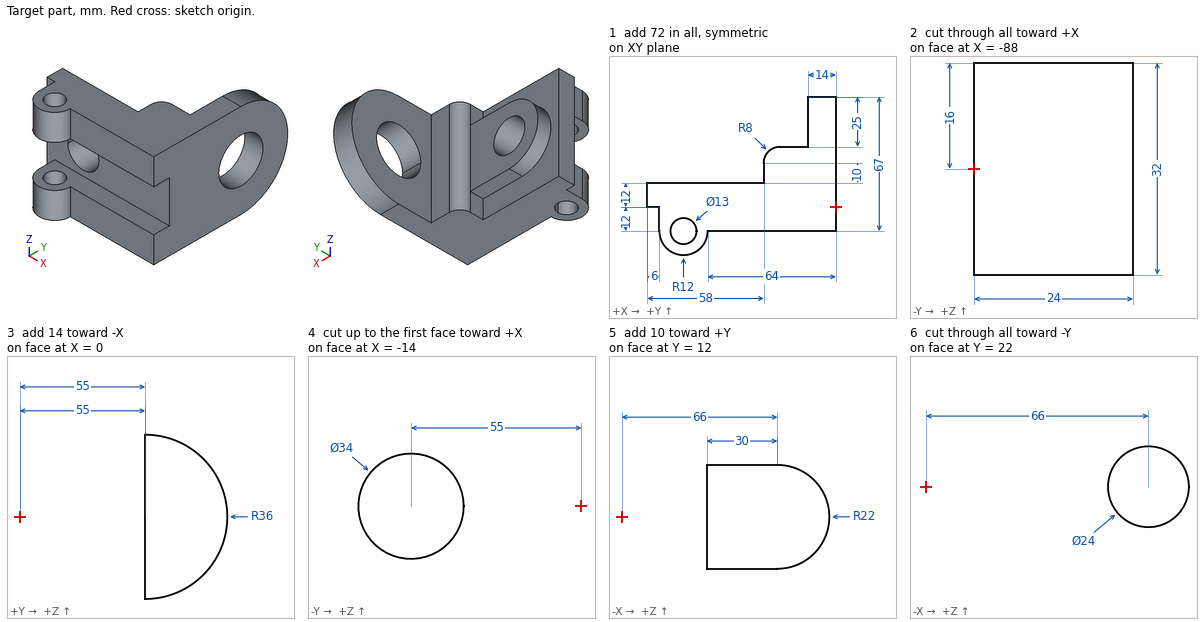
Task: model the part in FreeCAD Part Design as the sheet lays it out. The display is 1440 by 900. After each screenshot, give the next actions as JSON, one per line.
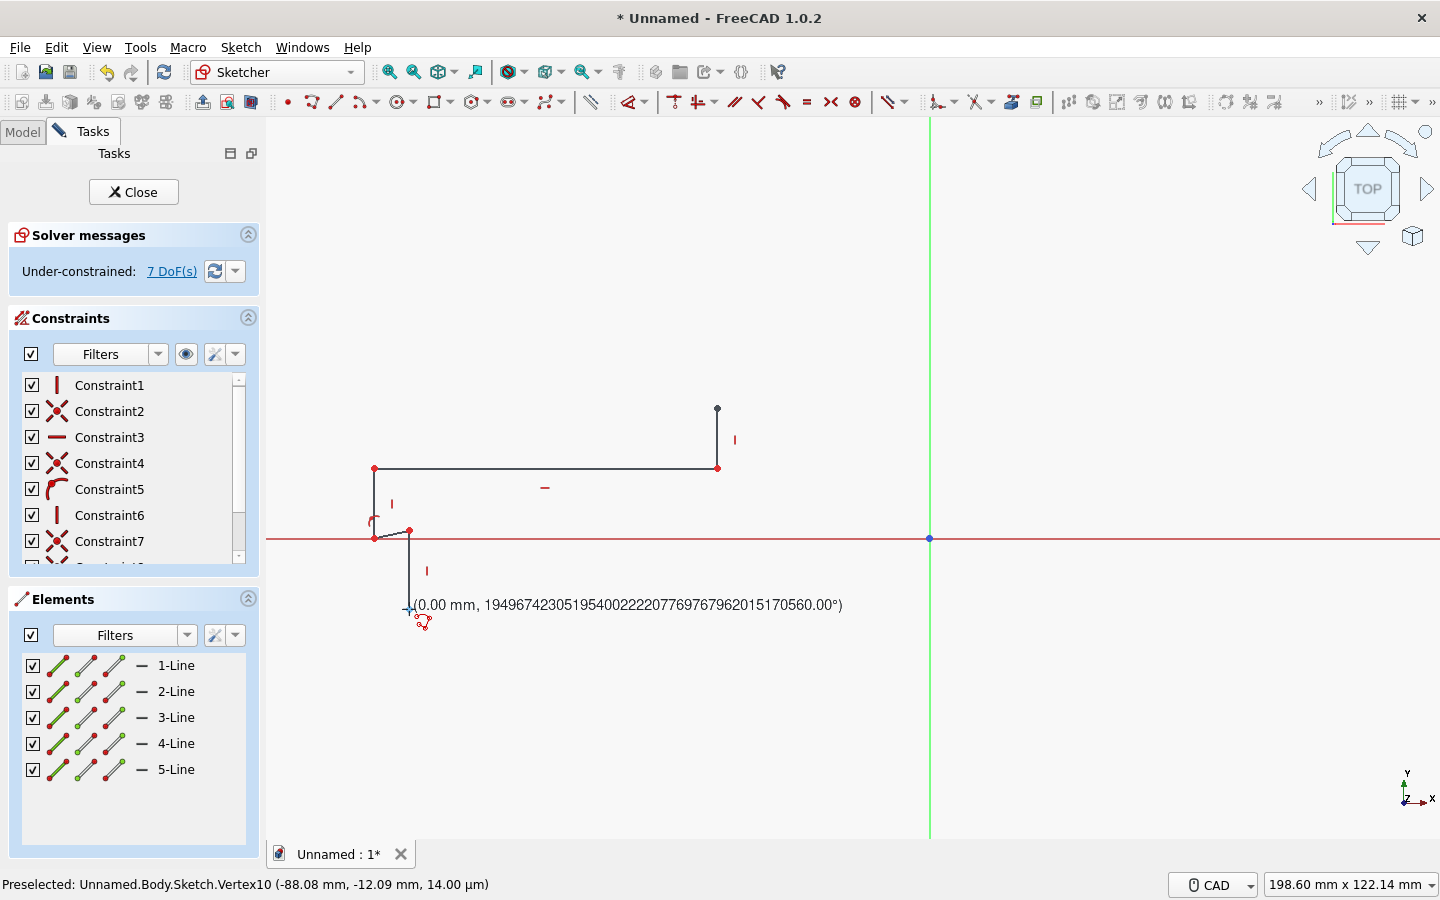
{"action": "left_click", "coordinate": [551, 609]}
{"action": "left_click", "coordinate": [930, 609]}
{"action": "left_click", "coordinate": [921, 213]}
{"action": "left_click", "coordinate": [847, 213]}
{"action": "left_click", "coordinate": [847, 361]}
{"action": "left_click", "coordinate": [764, 361]}
{"action": "right_click", "coordinate": [764, 361]}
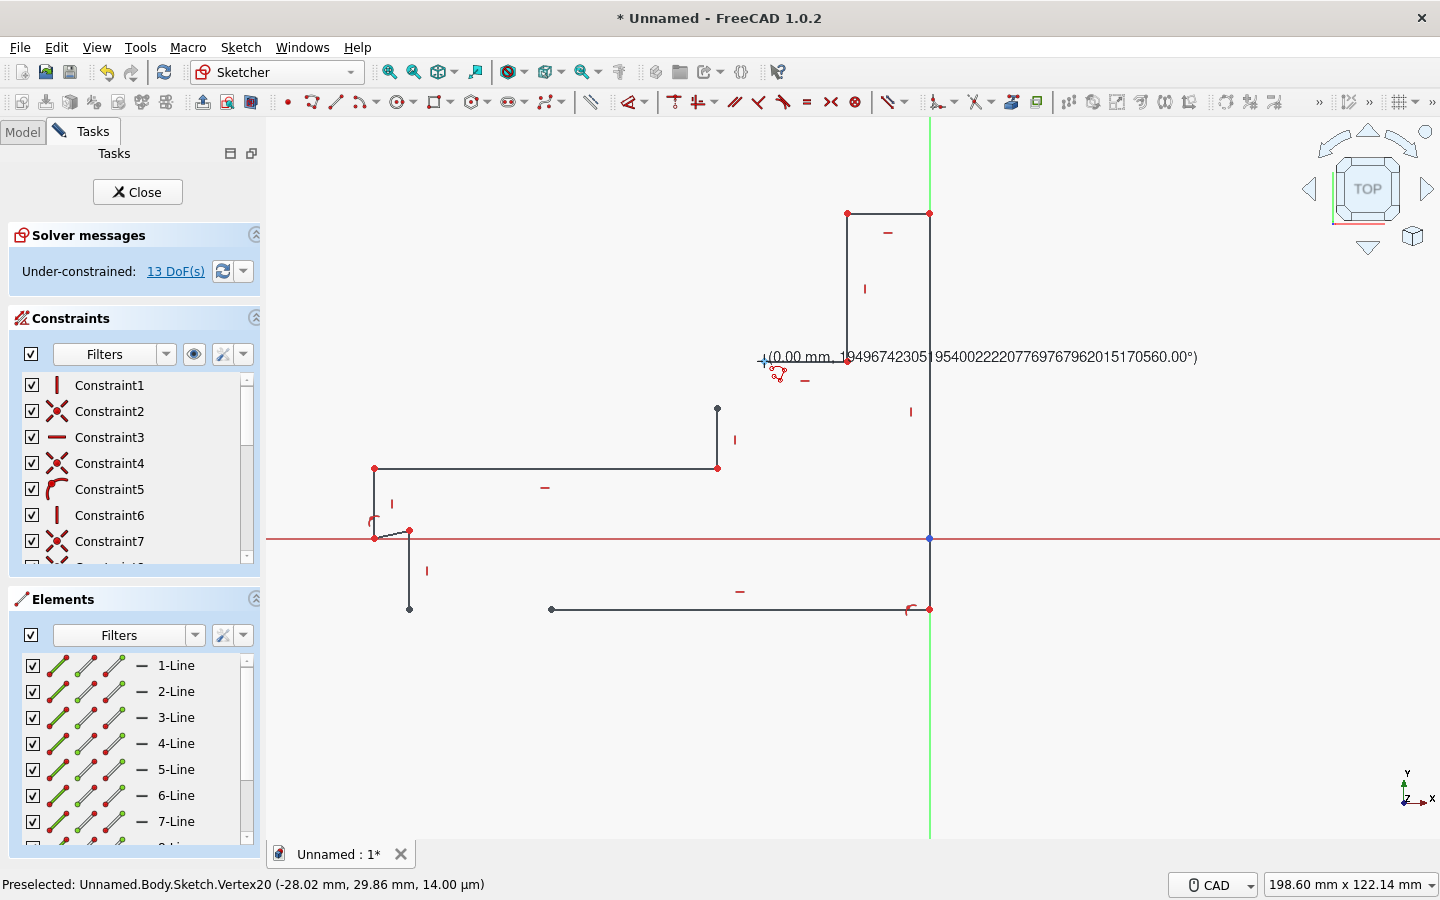
{"action": "left_click", "coordinate": [378, 102]}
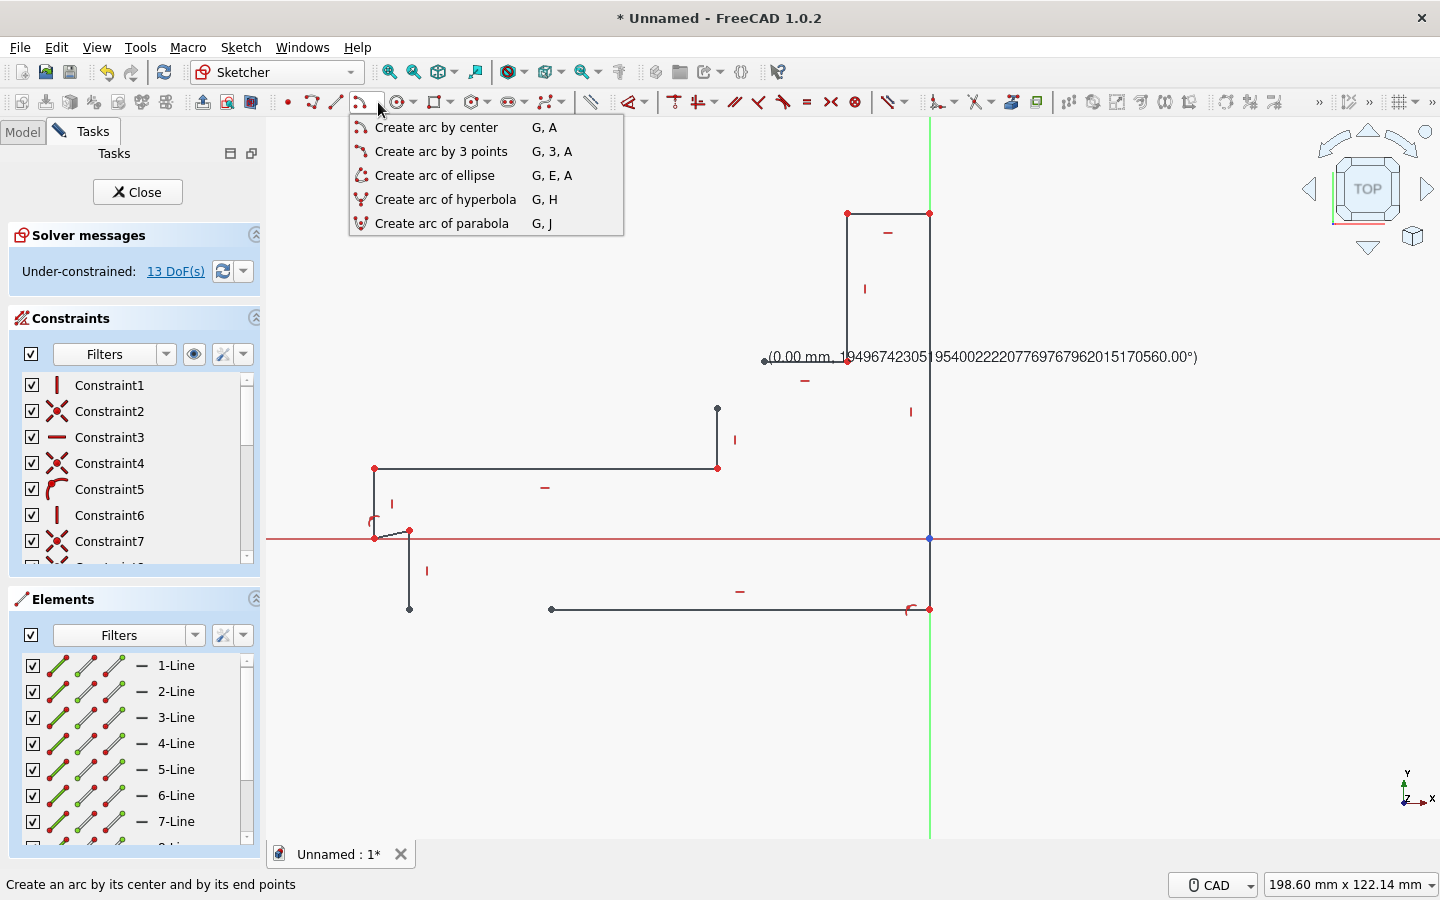
{"action": "left_click", "coordinate": [486, 151]}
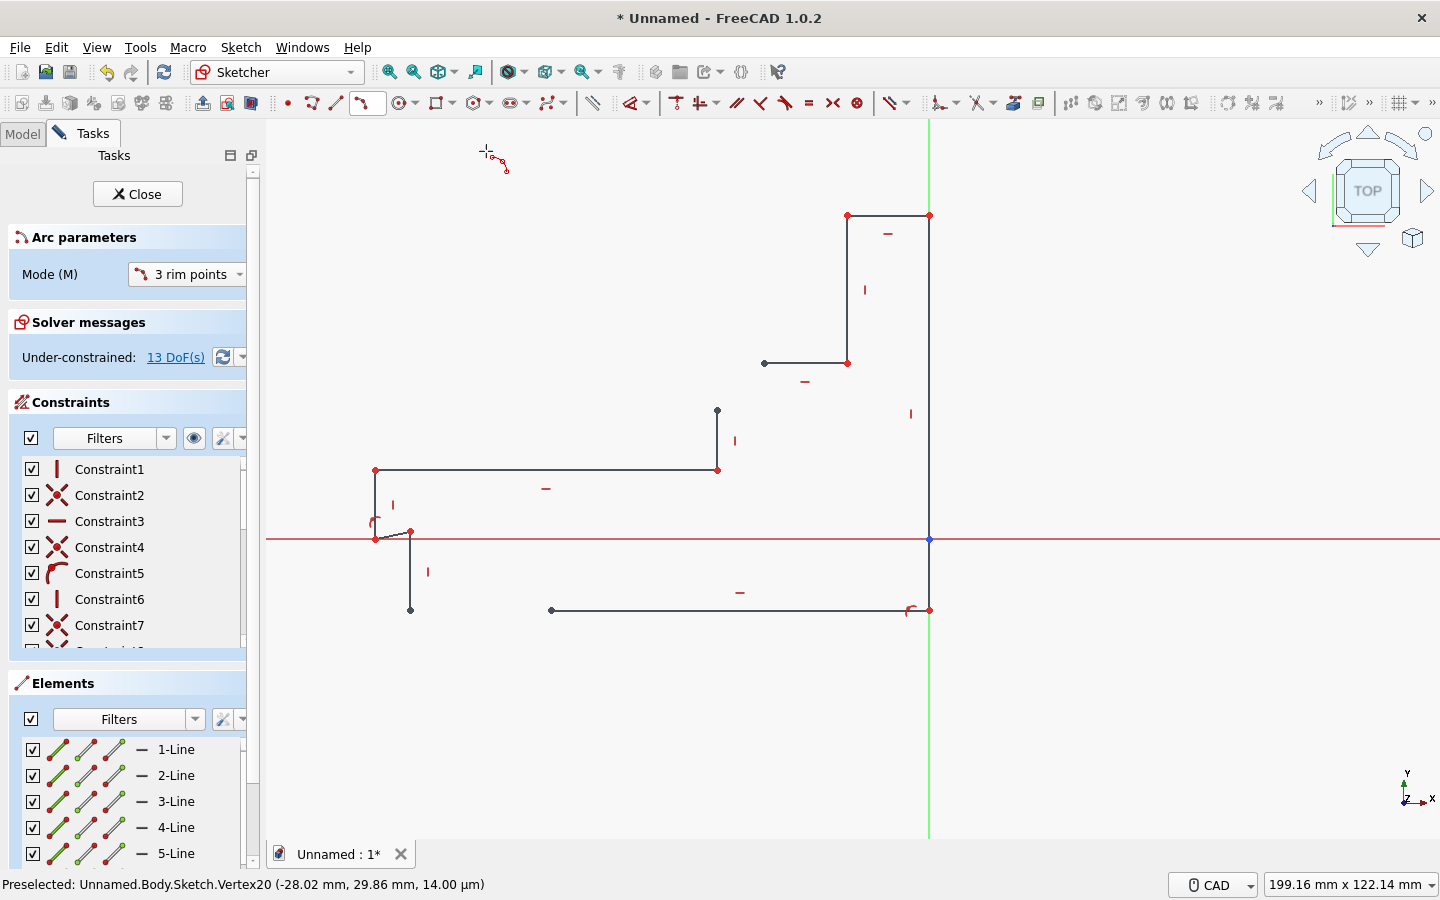
{"action": "left_click", "coordinate": [410, 611]}
{"action": "left_click", "coordinate": [552, 611]}
{"action": "left_click", "coordinate": [481, 681]}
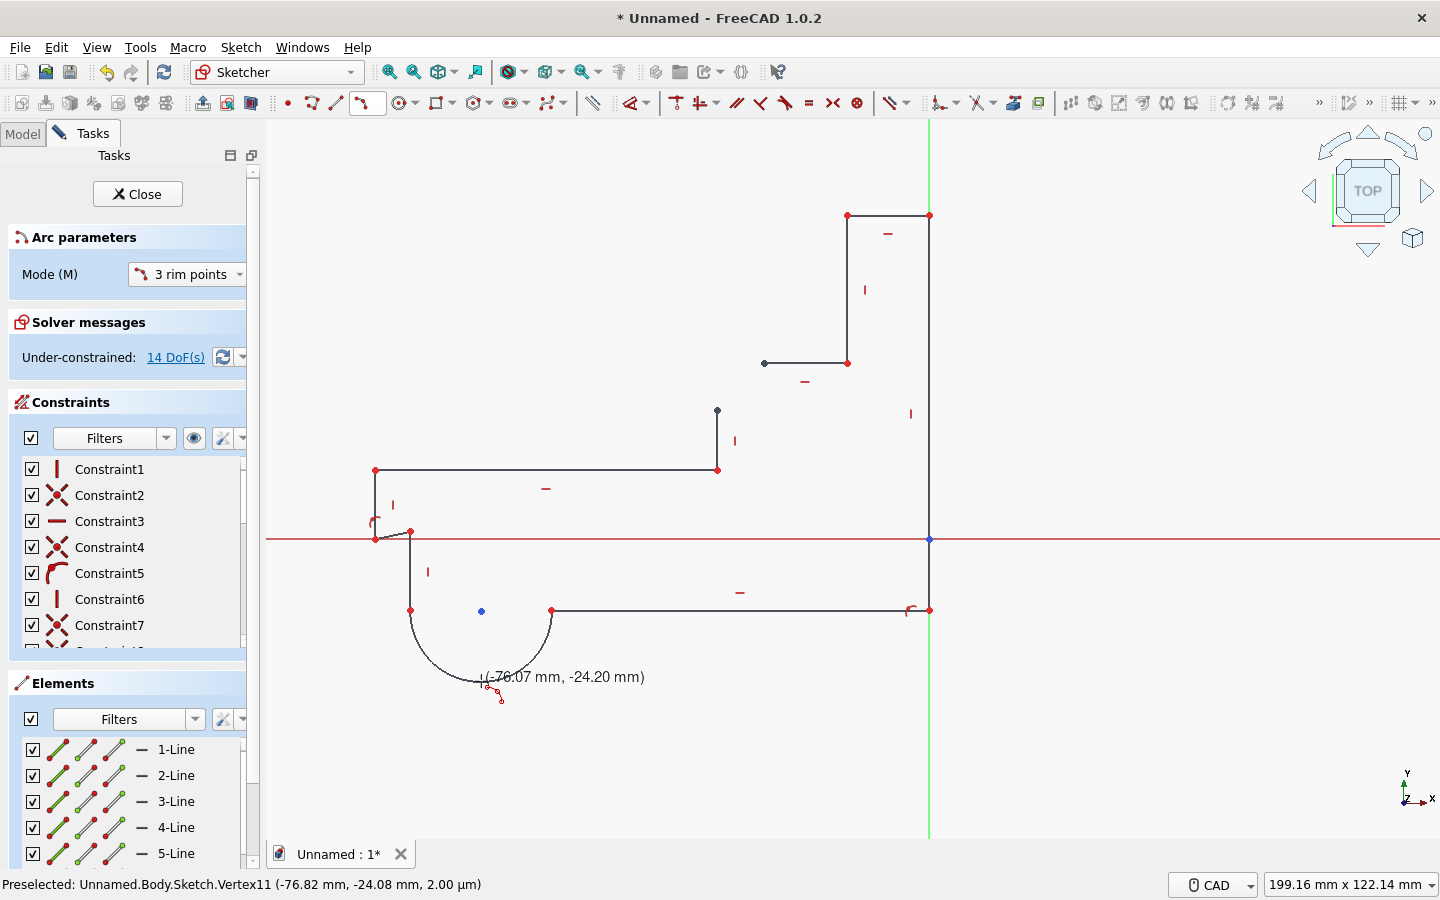
{"action": "left_click", "coordinate": [764, 363]}
{"action": "left_click", "coordinate": [717, 410]}
{"action": "left_click", "coordinate": [731, 376]}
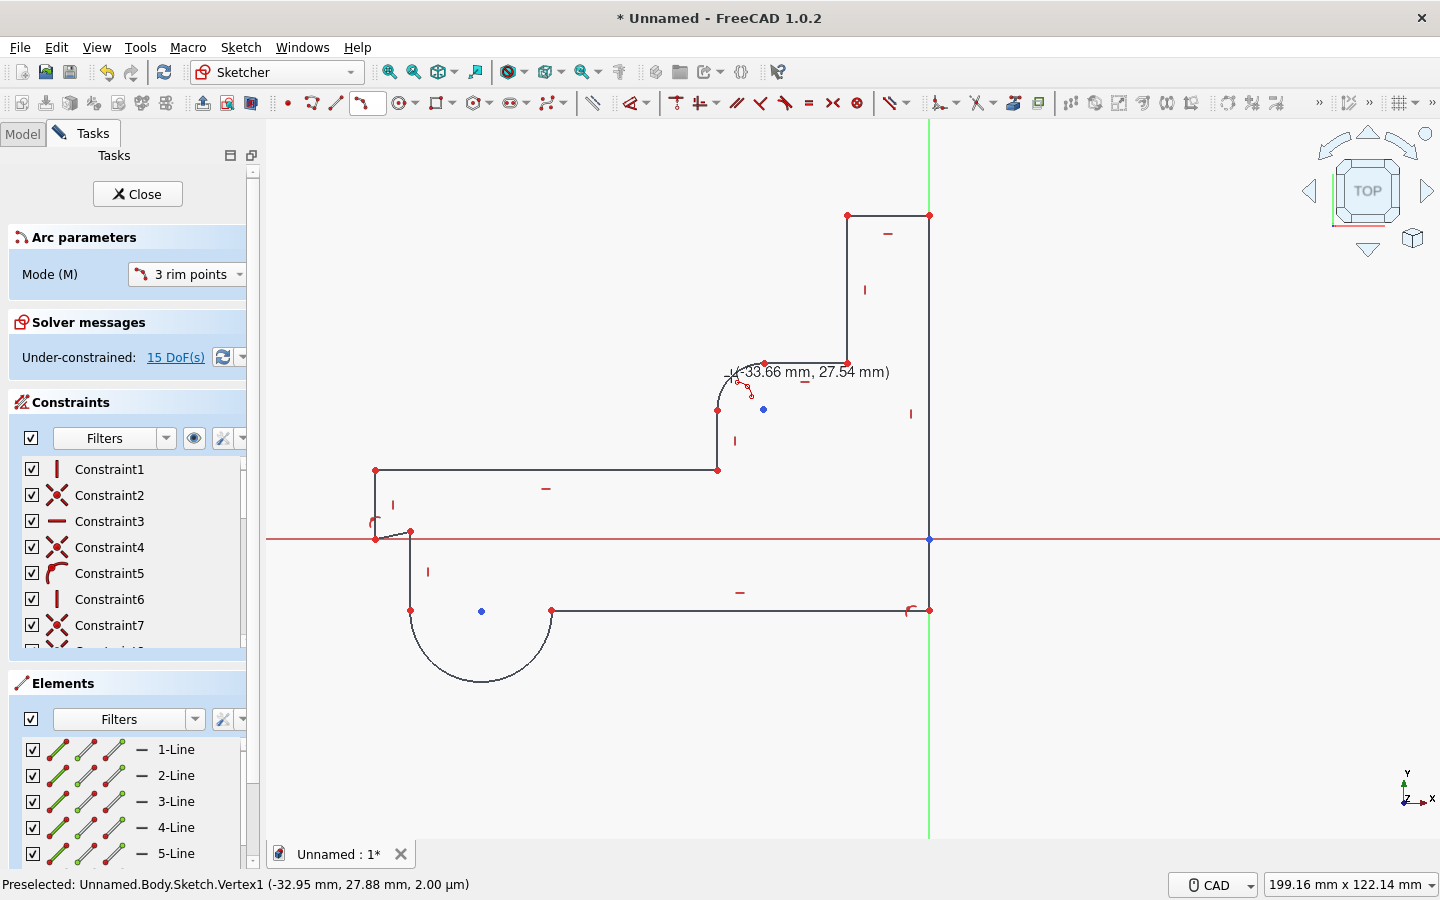
{"action": "left_click", "coordinate": [400, 104]}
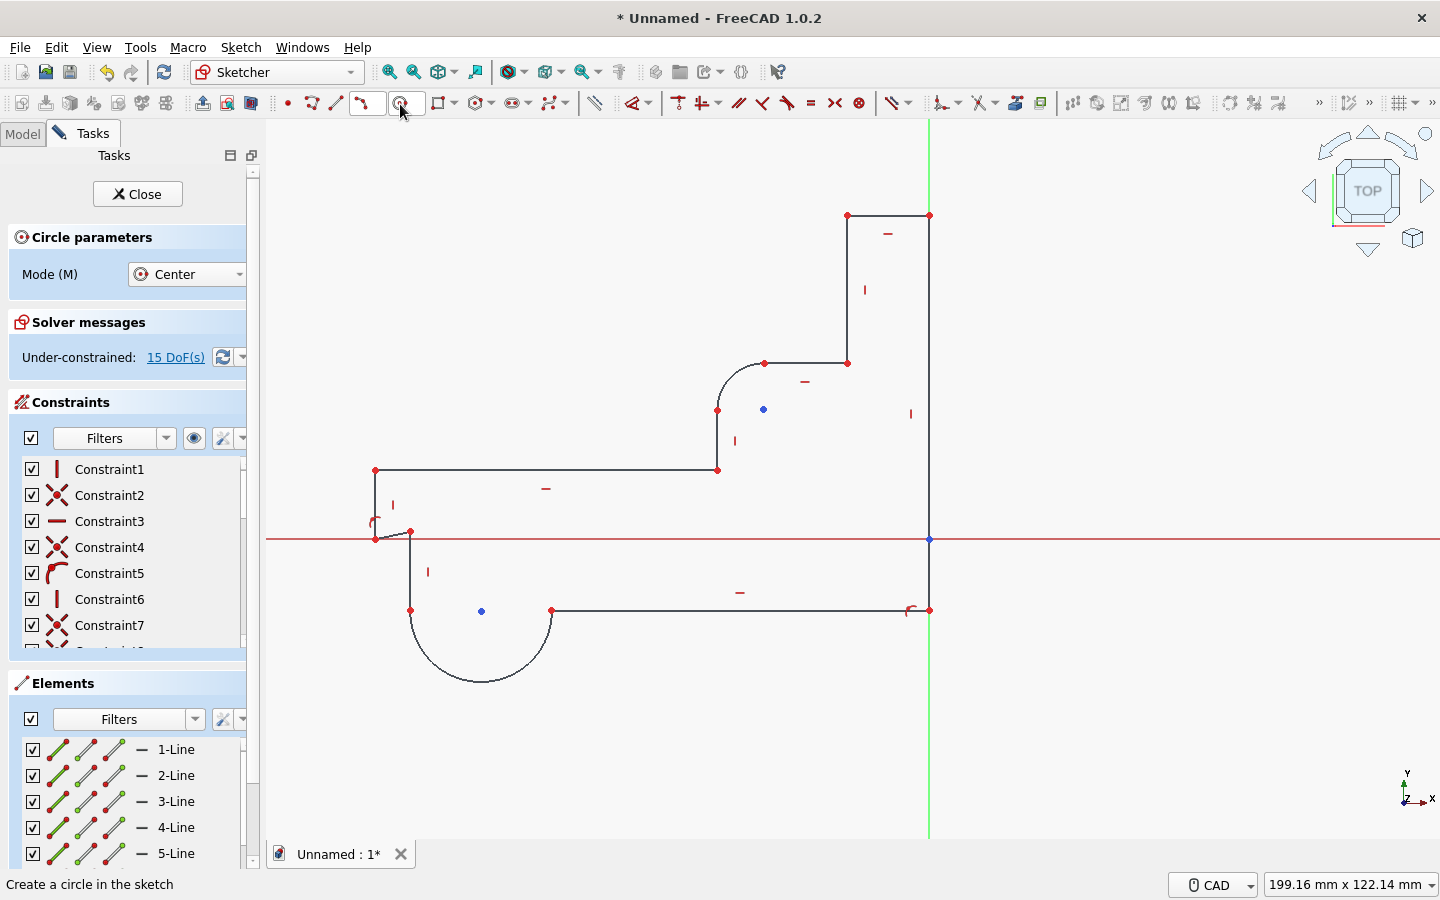
{"action": "left_click", "coordinate": [481, 610]}
{"action": "mouse_move", "coordinate": [509, 583]}